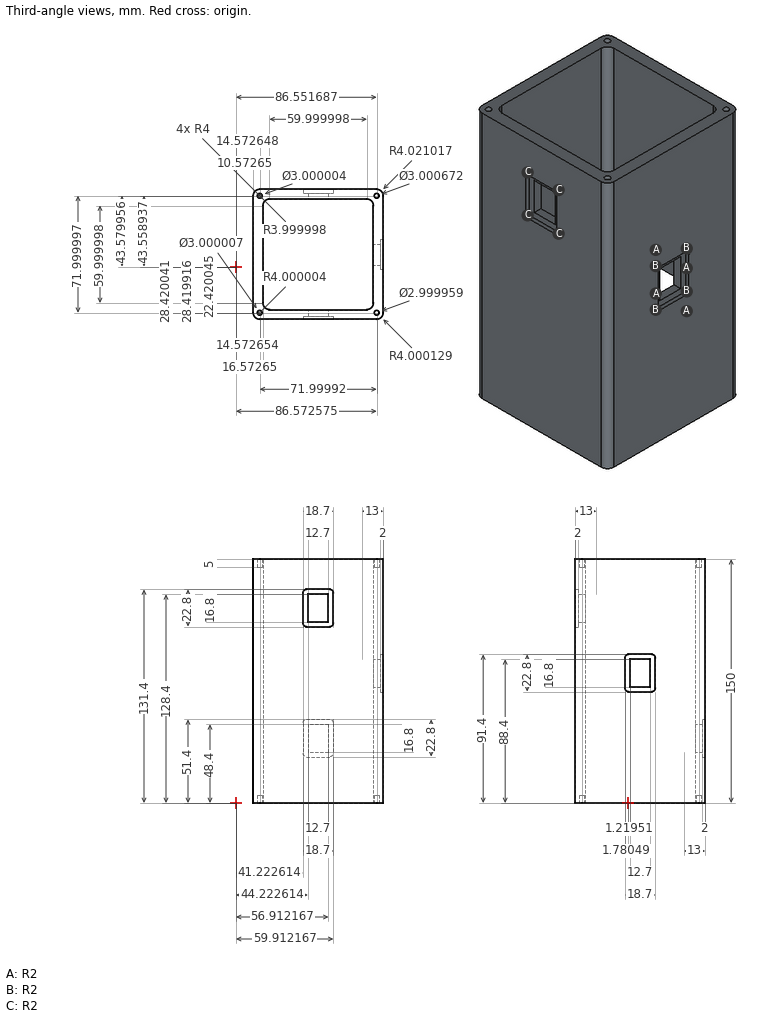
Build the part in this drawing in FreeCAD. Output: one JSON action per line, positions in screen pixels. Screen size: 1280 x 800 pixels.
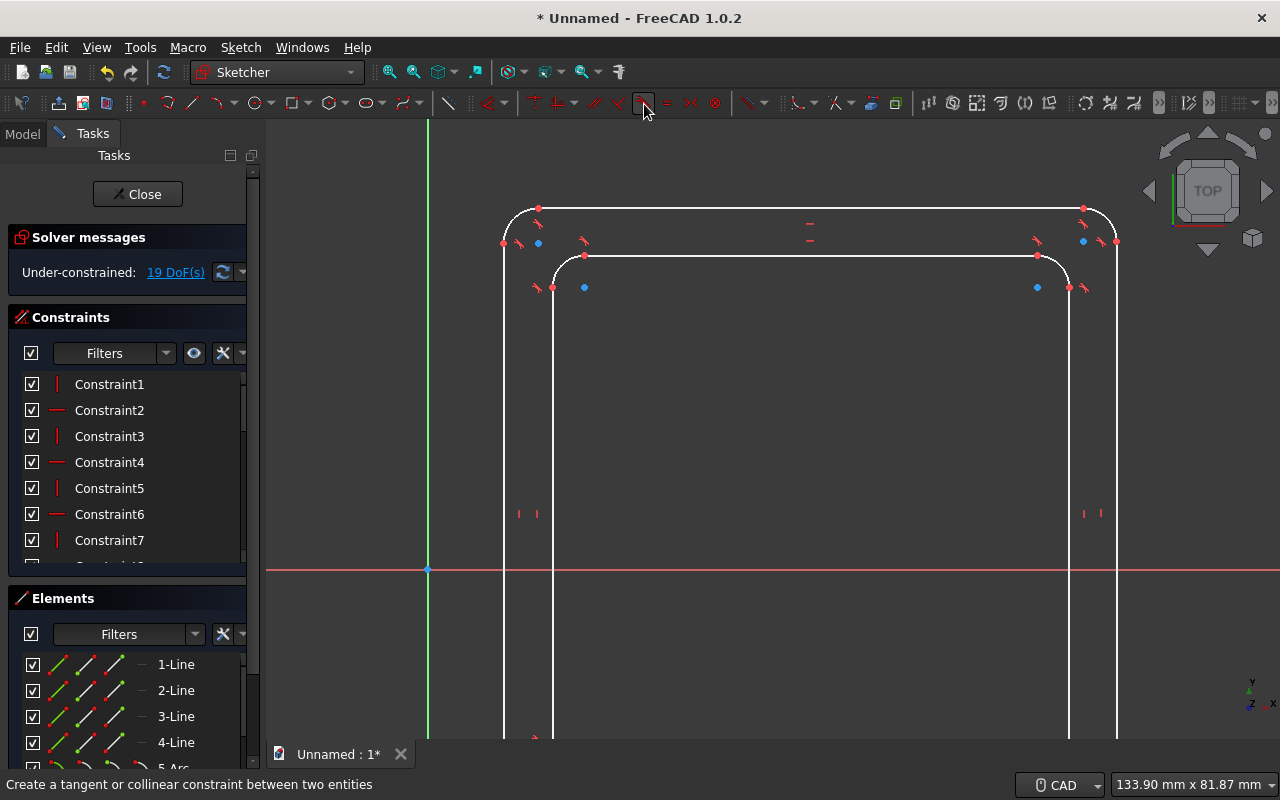
{"action": "left_click", "coordinate": [1069, 423]}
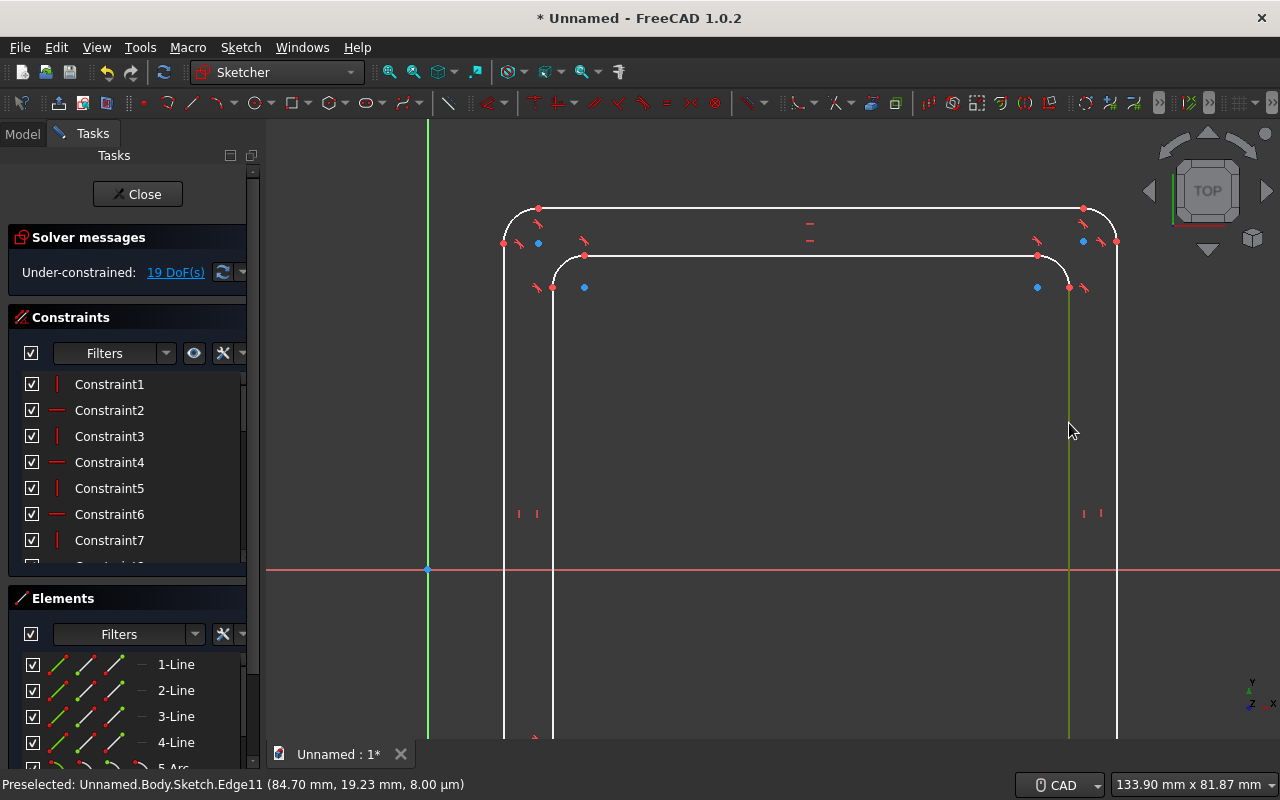
{"action": "scroll", "coordinate": [570, 260], "scroll_direction": "down", "scroll_amount": 2}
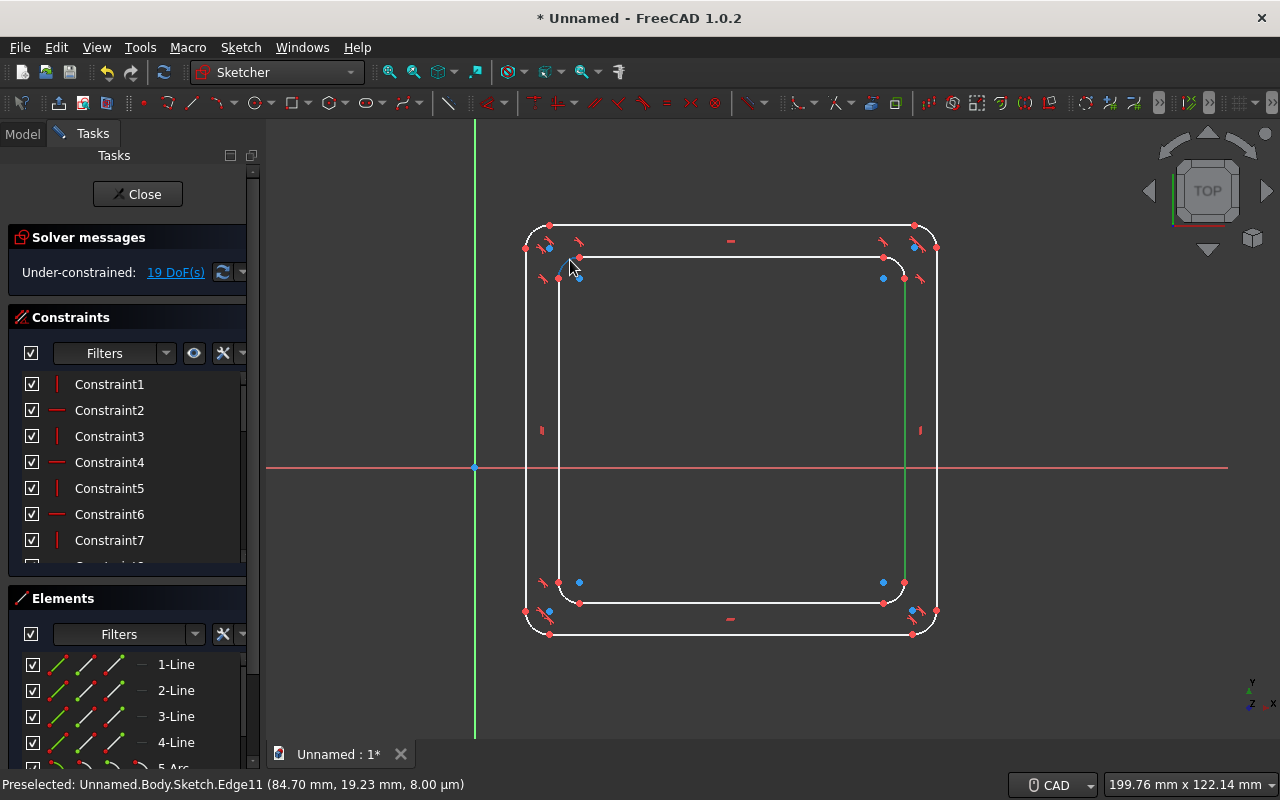
{"action": "scroll", "coordinate": [893, 601], "scroll_direction": "up", "scroll_amount": 2}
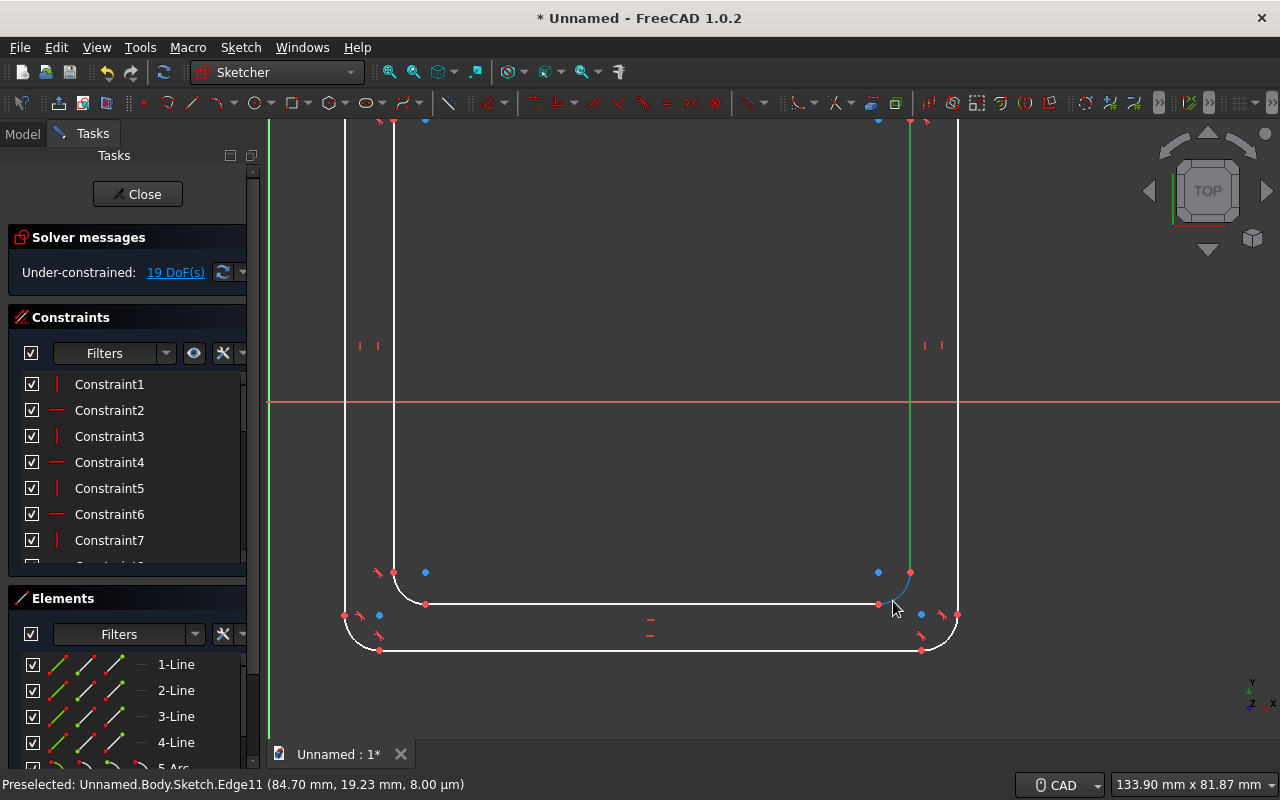
{"action": "left_click", "coordinate": [893, 601]}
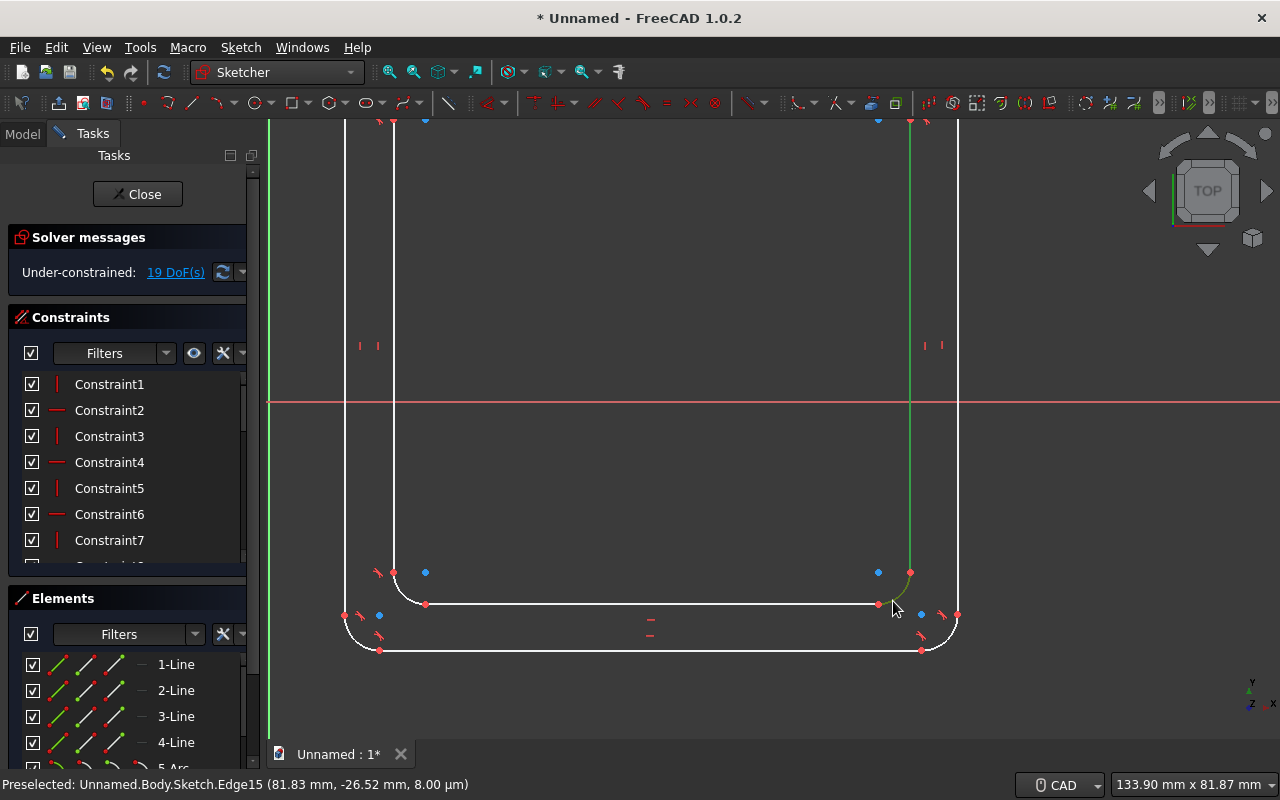
{"action": "left_click", "coordinate": [644, 104]}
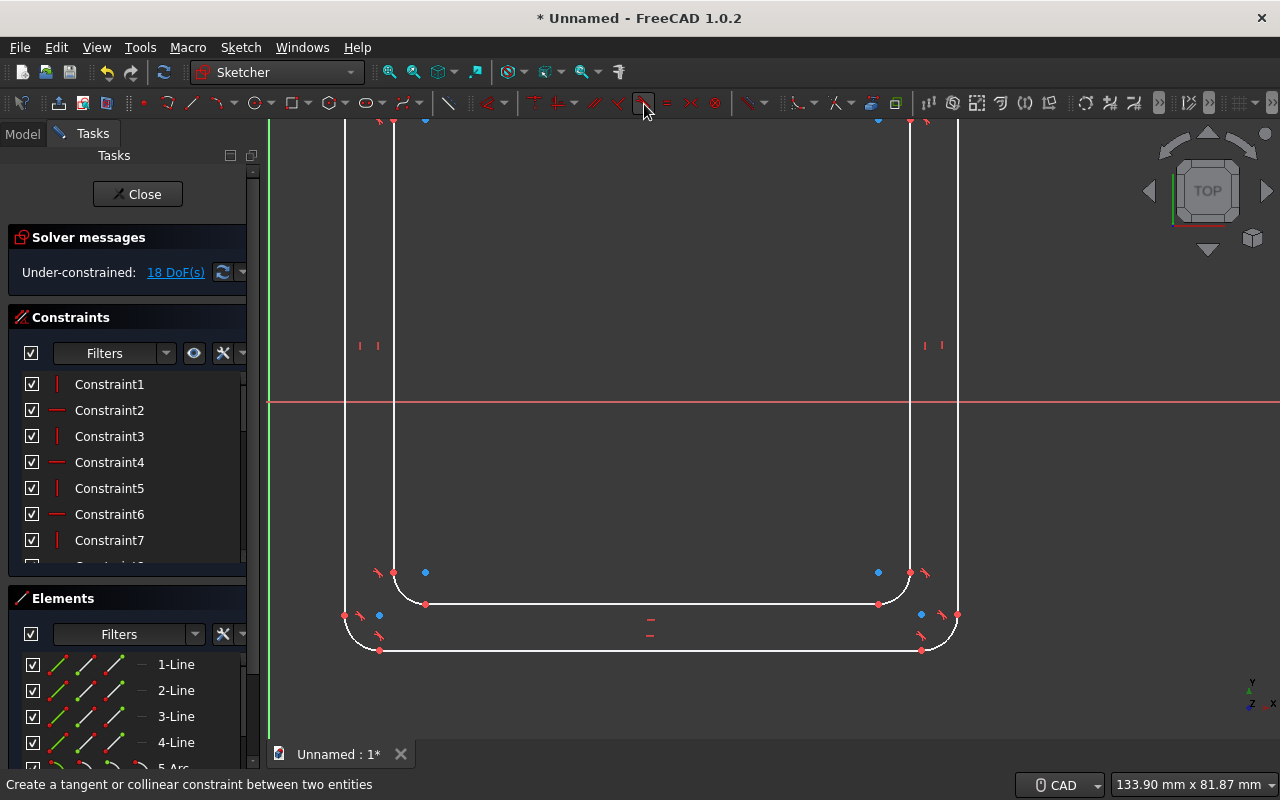
{"action": "left_click", "coordinate": [743, 604]}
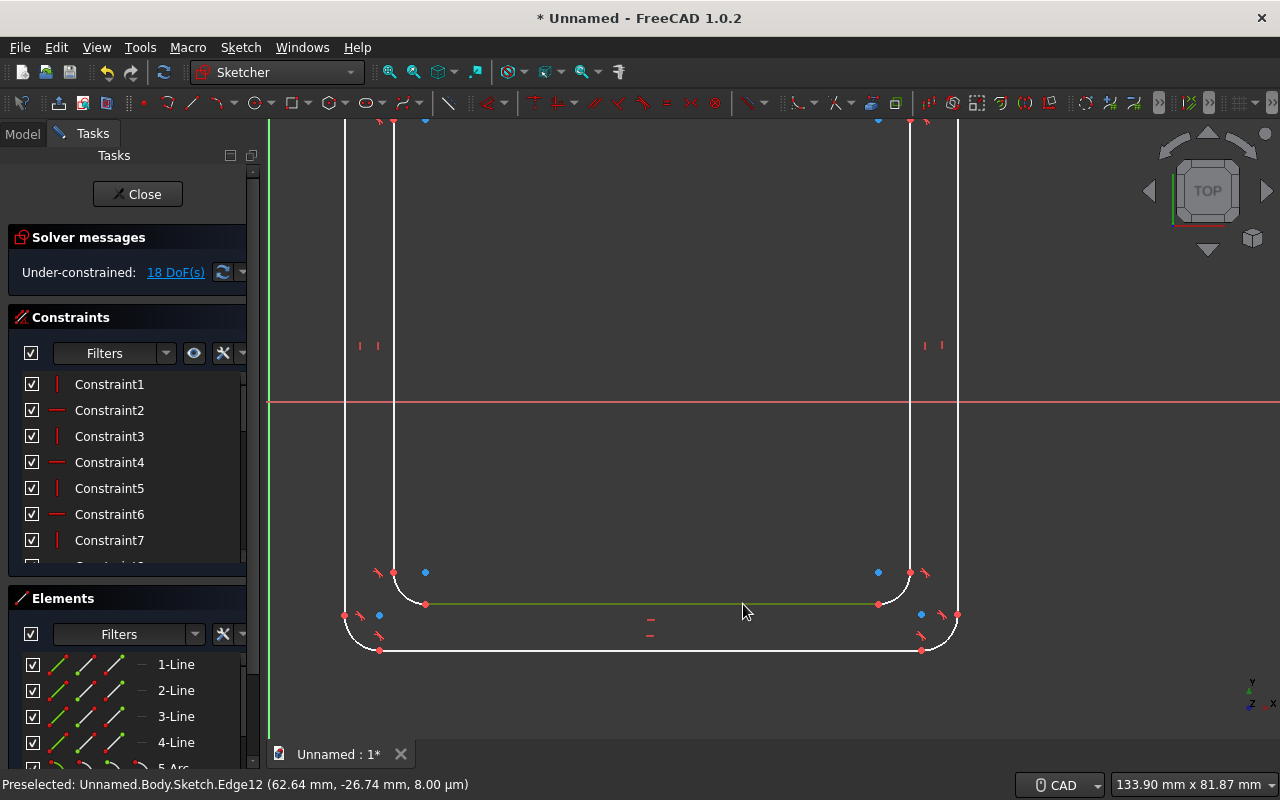
{"action": "left_click", "coordinate": [893, 601]}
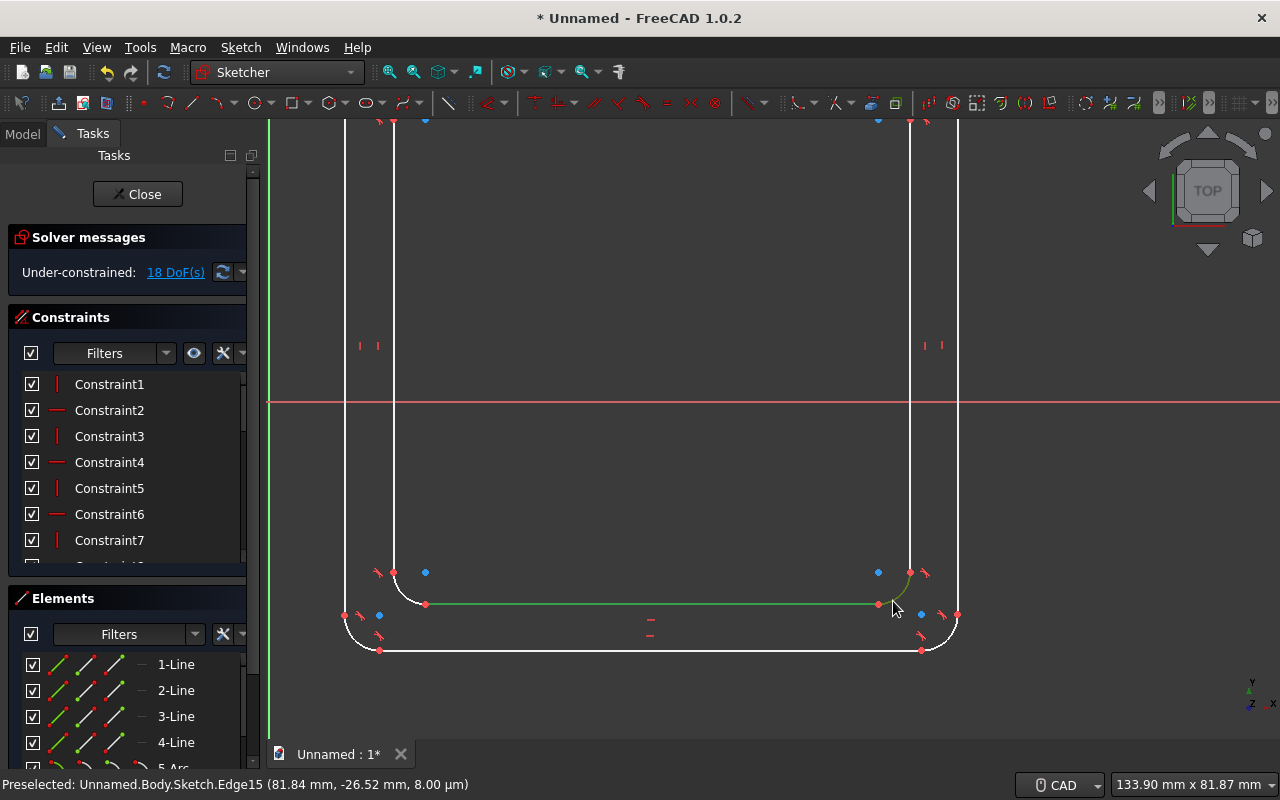
{"action": "left_click", "coordinate": [644, 104]}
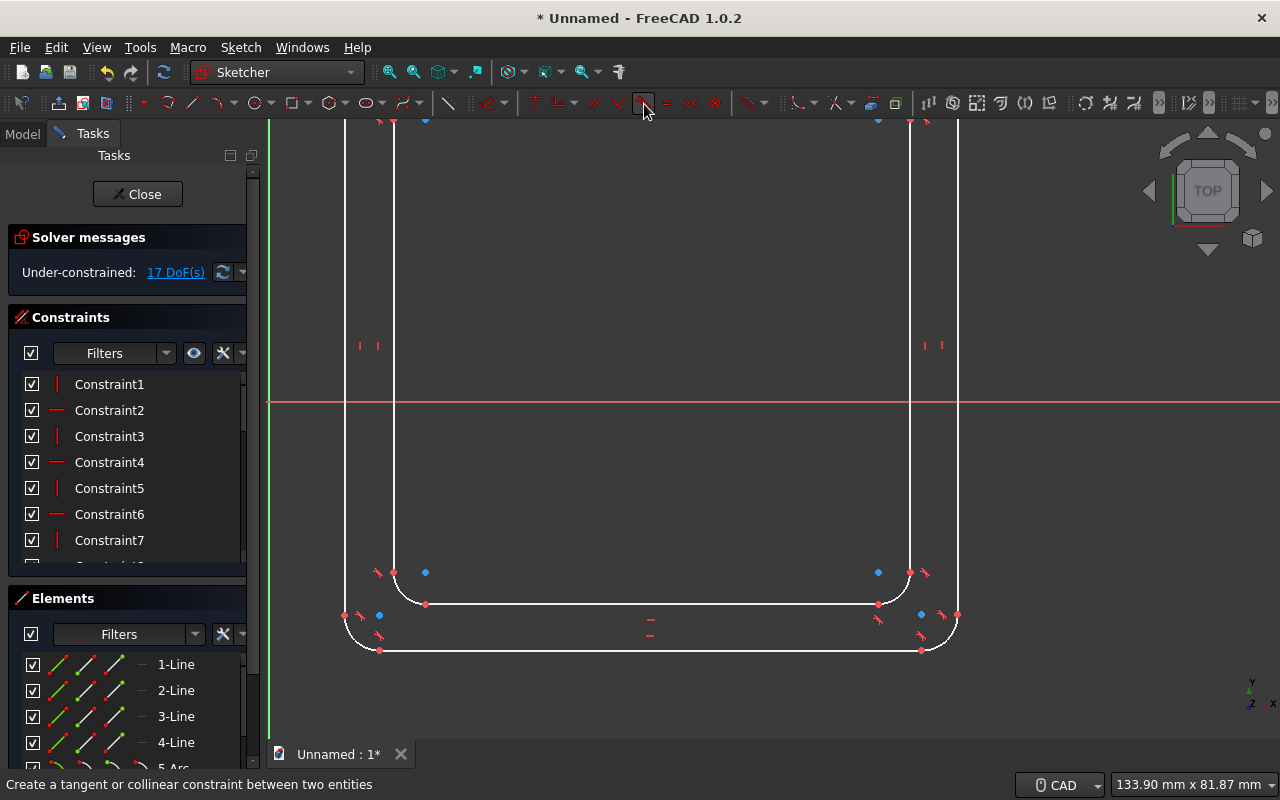
{"action": "left_click", "coordinate": [742, 604]}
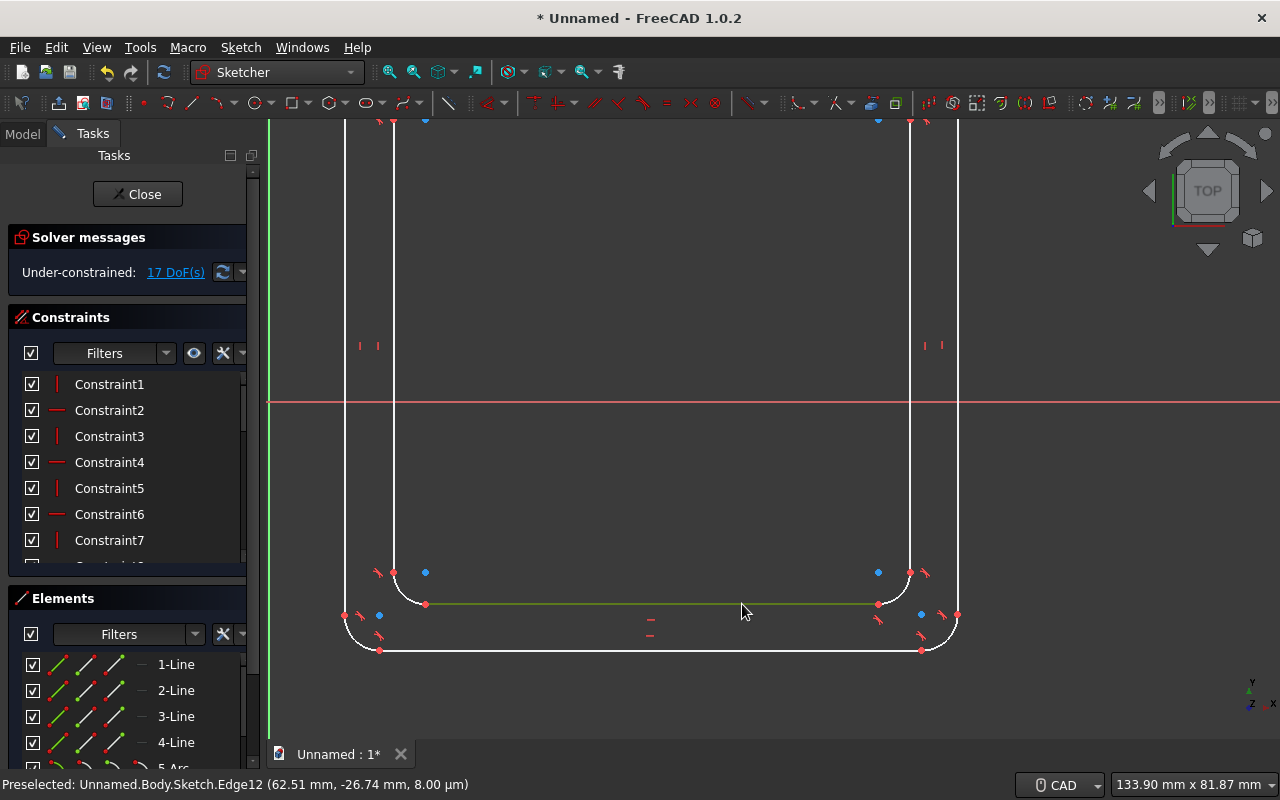
{"action": "left_click", "coordinate": [397, 587]}